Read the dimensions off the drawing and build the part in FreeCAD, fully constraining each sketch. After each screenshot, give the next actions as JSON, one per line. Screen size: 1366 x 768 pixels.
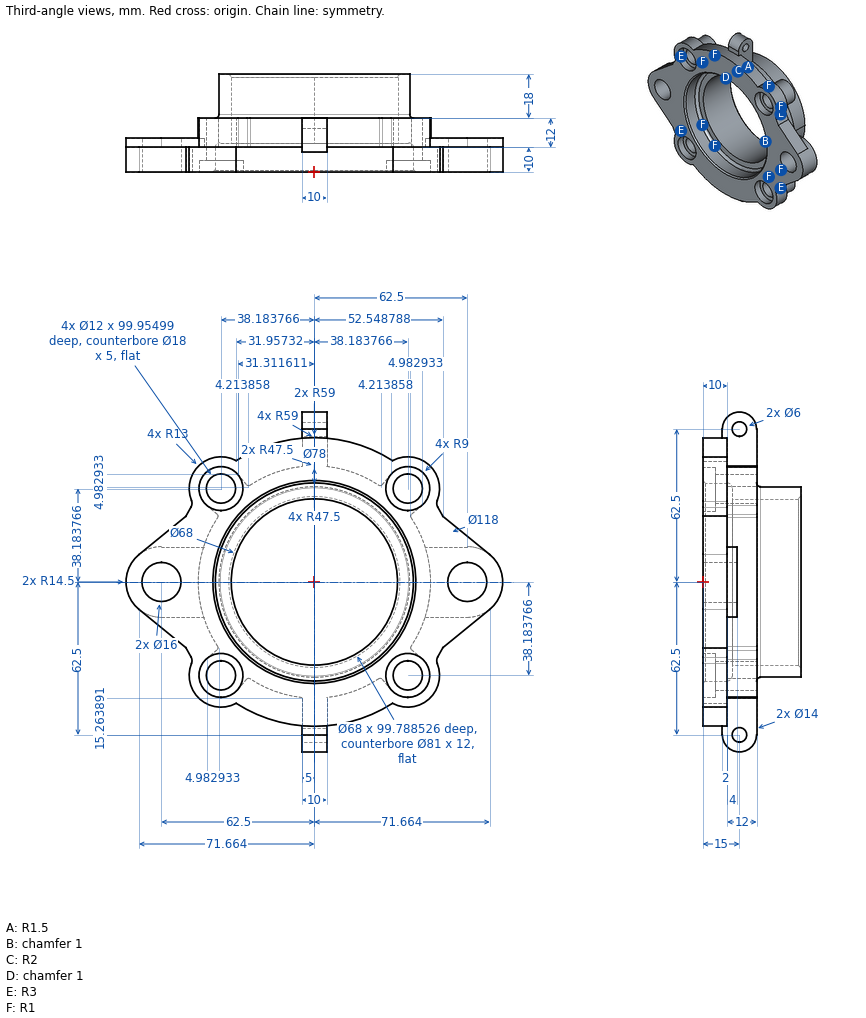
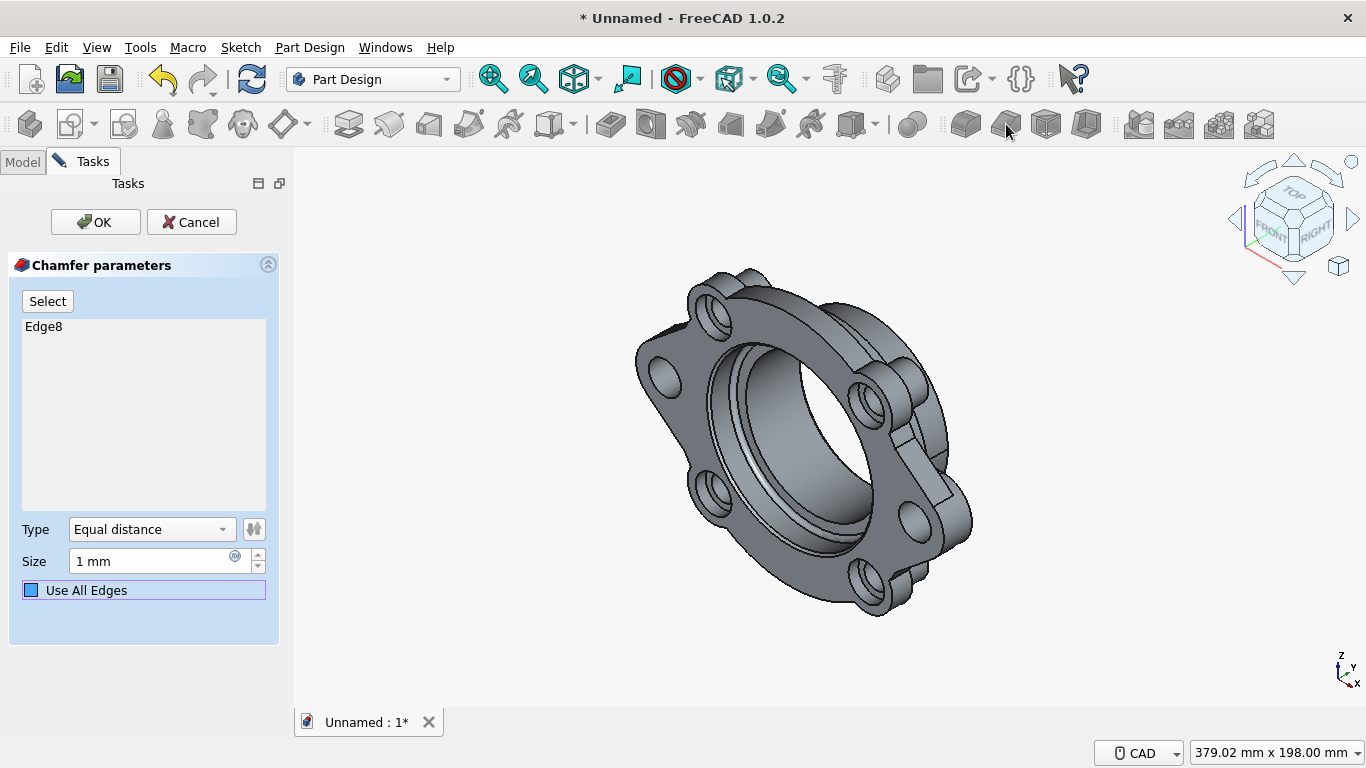
{"action": "left_click", "coordinate": [96, 222]}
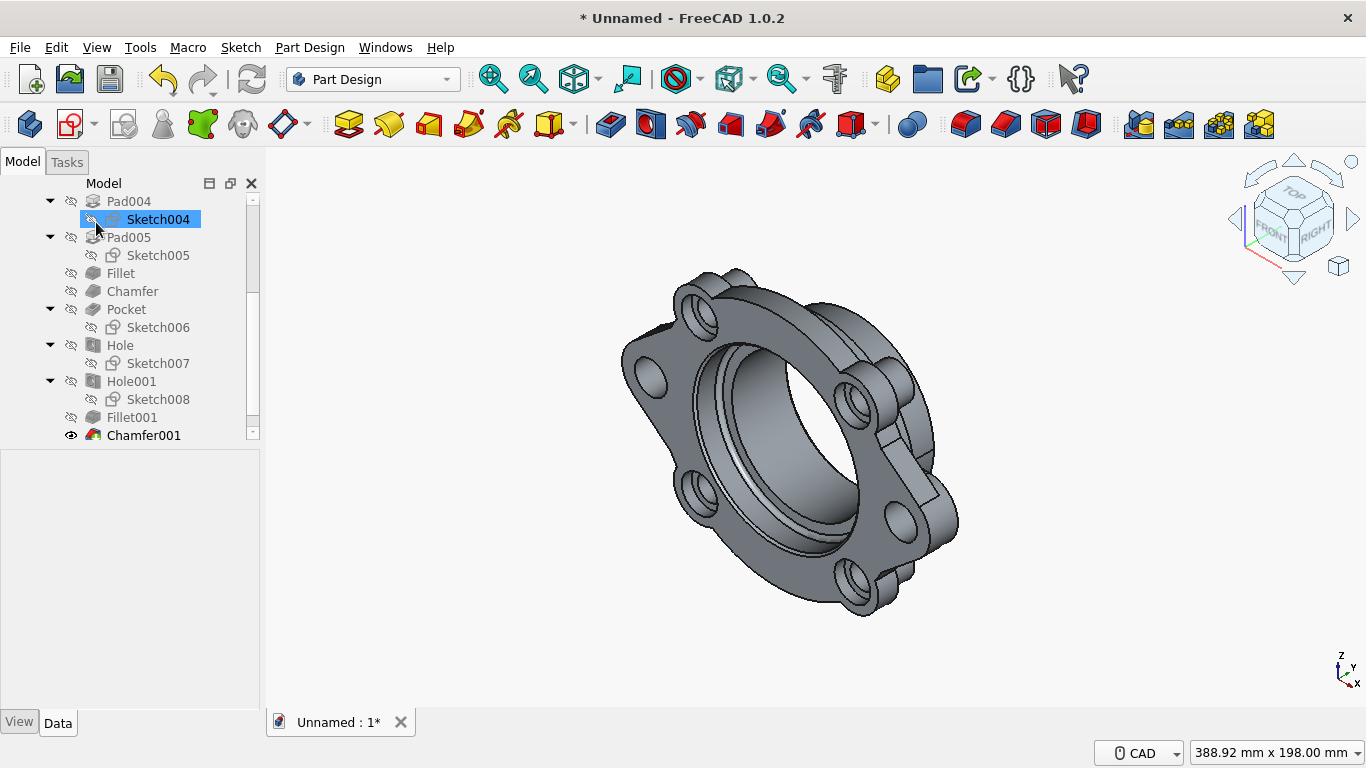
{"action": "key", "text": "4"}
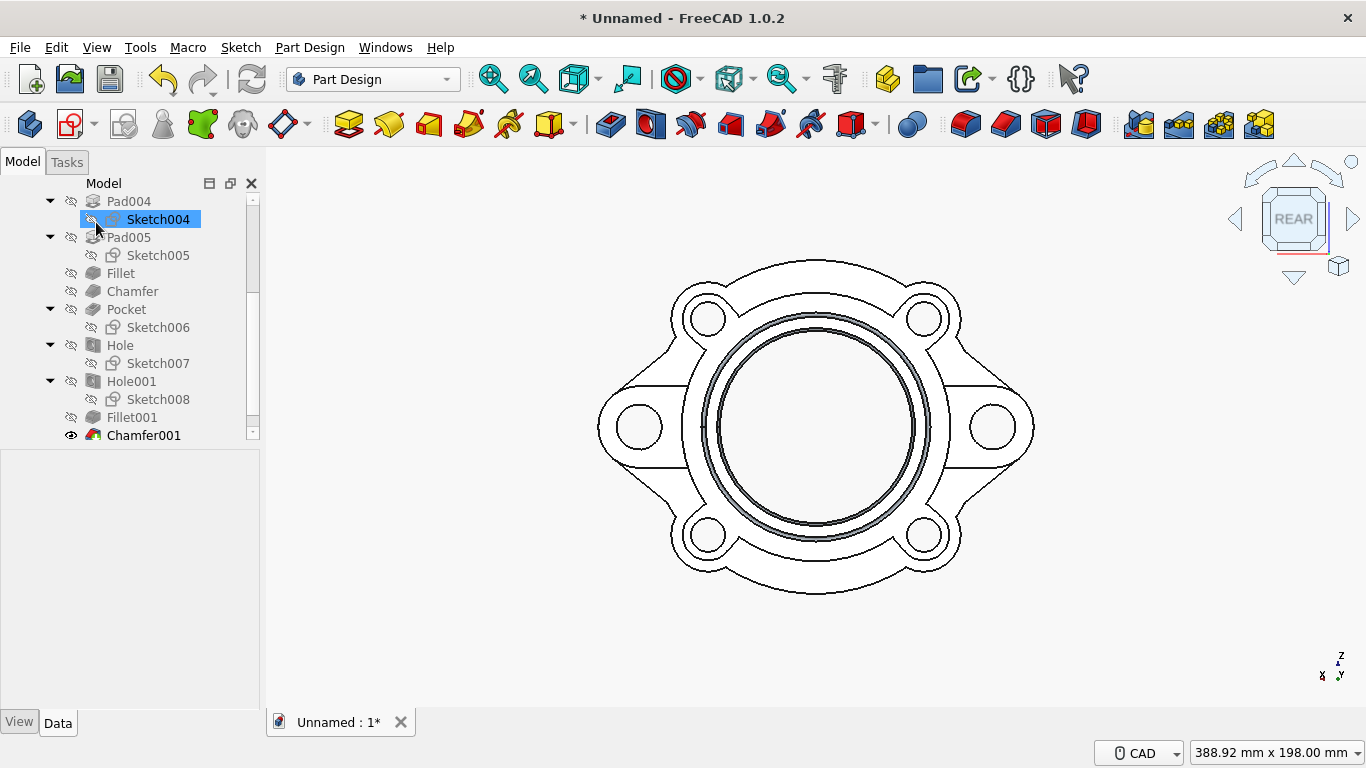
{"action": "left_click", "coordinate": [758, 288]}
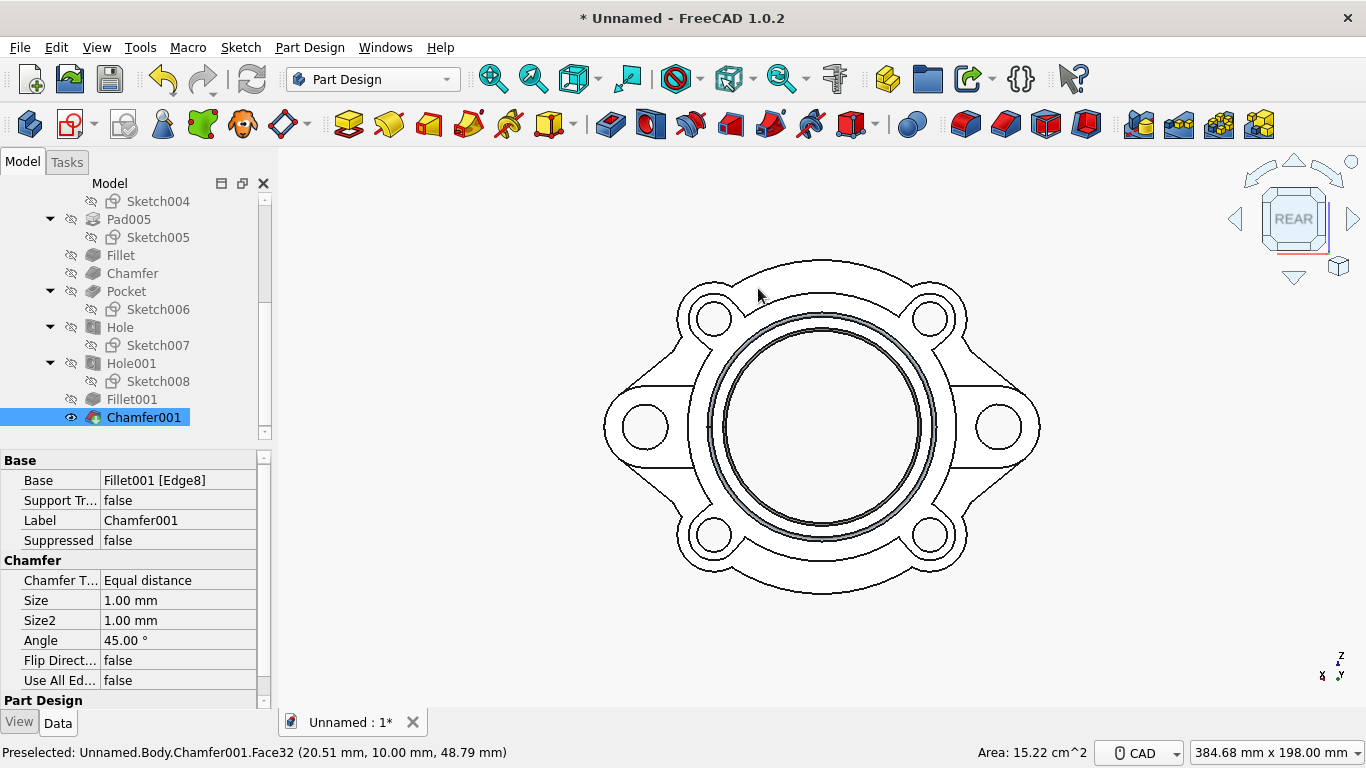
{"action": "left_click", "coordinate": [70, 124]}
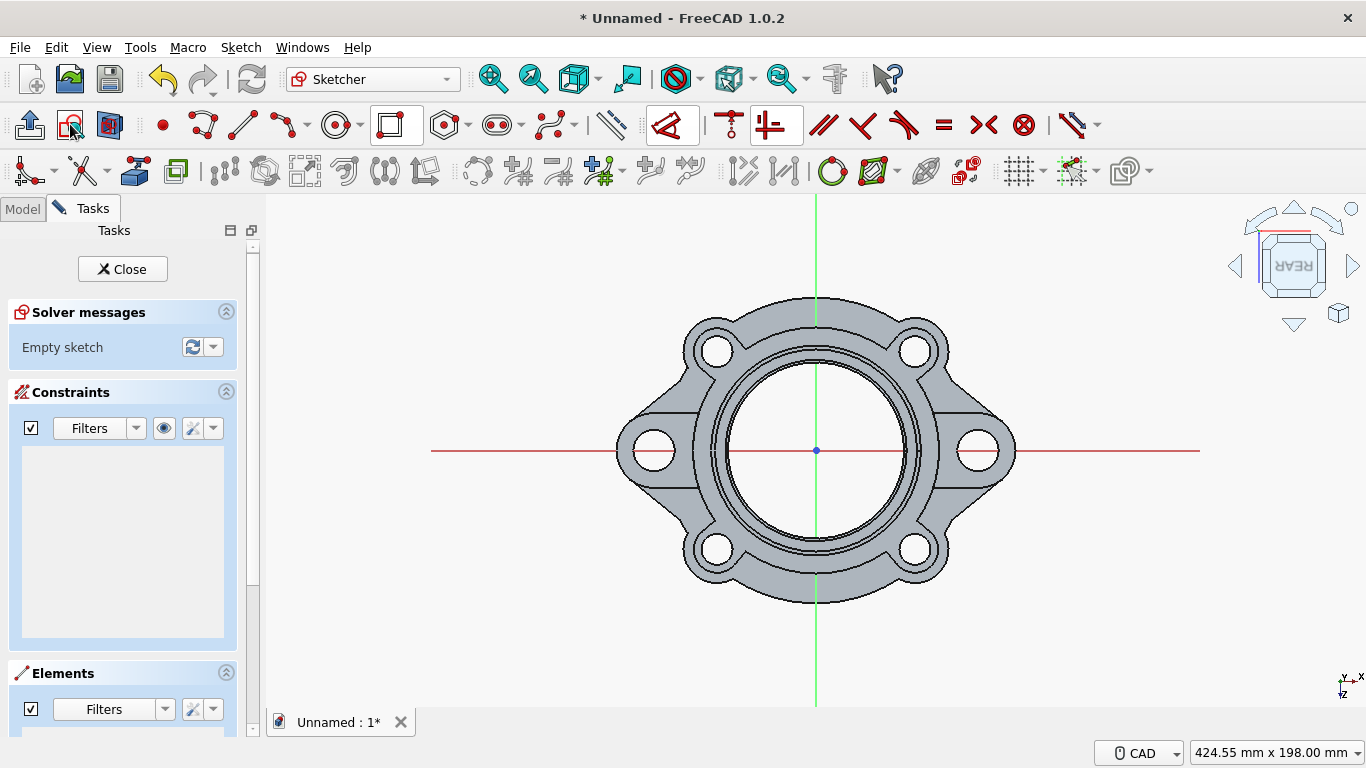
{"action": "left_click", "coordinate": [110, 126]}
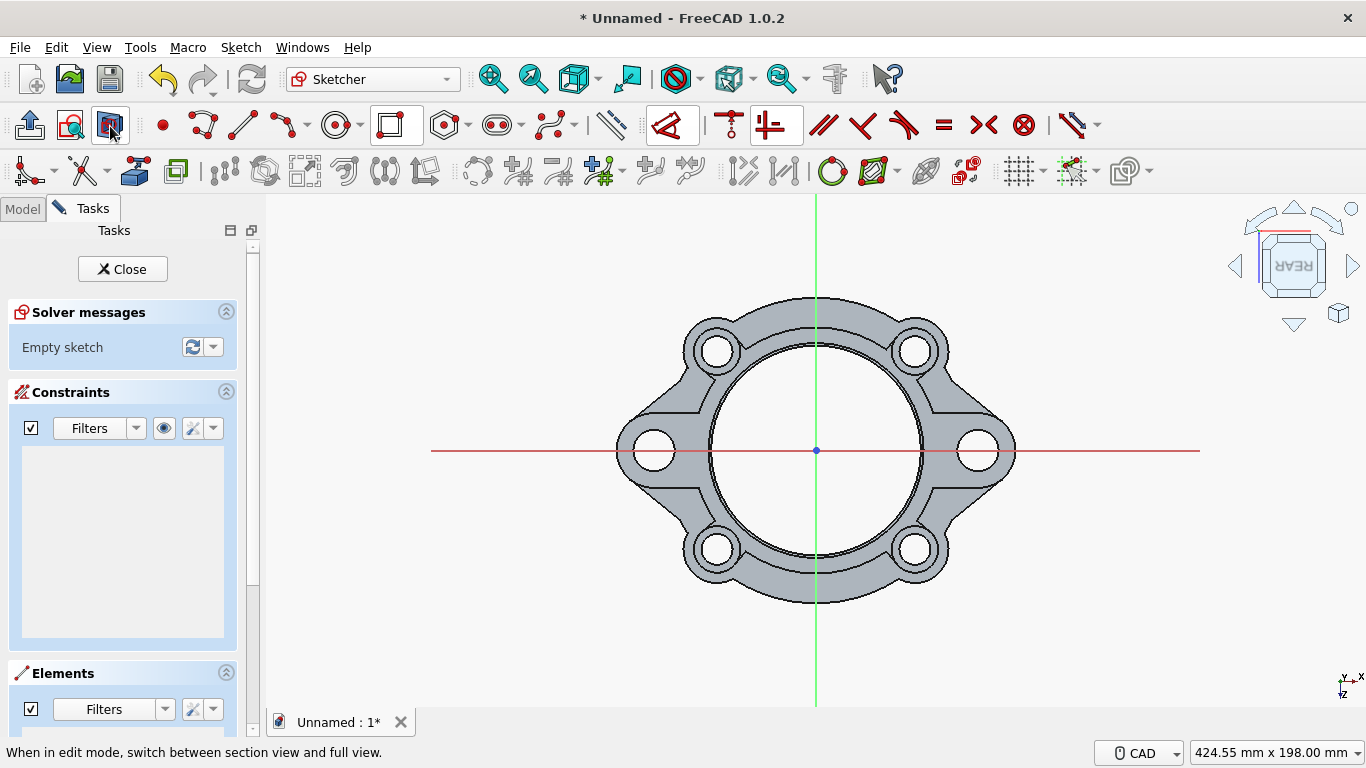
{"action": "left_click", "coordinate": [390, 126]}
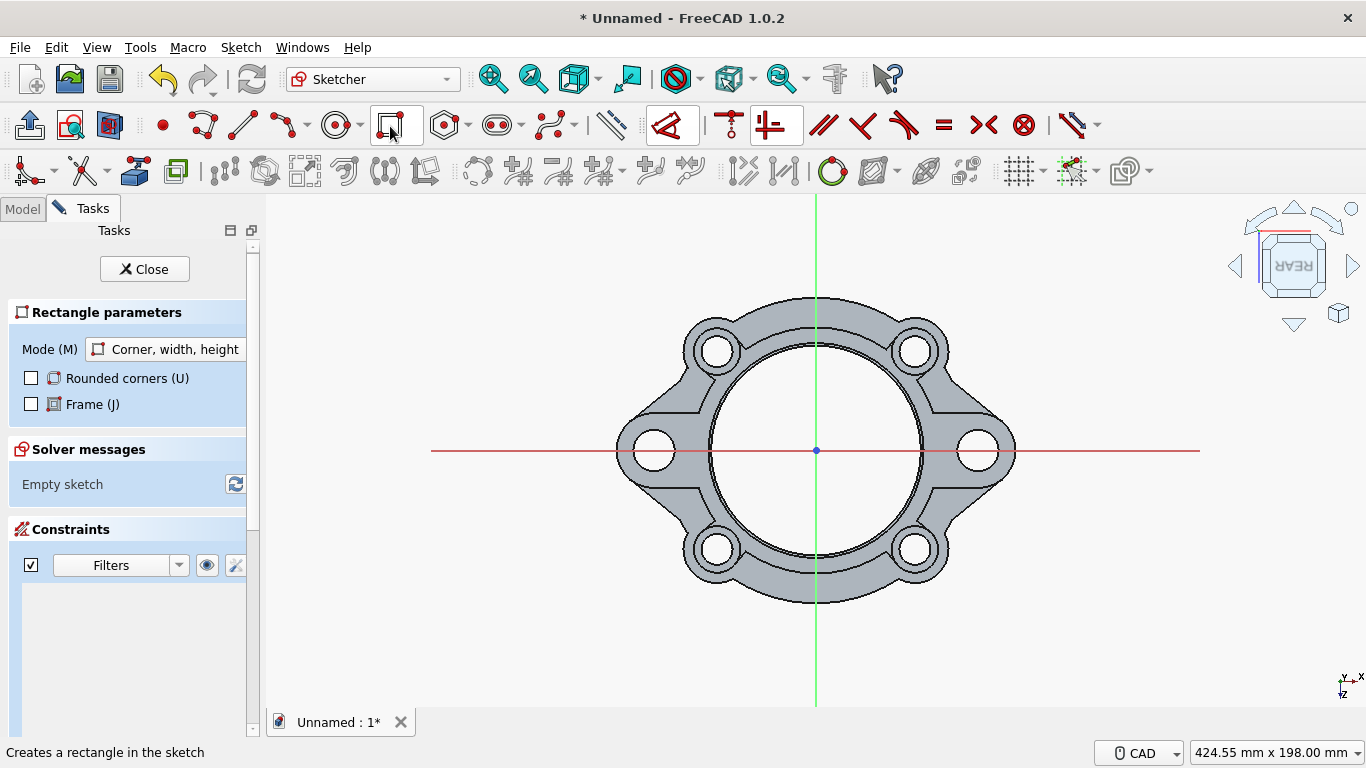
{"action": "scroll", "coordinate": [803, 289], "scroll_direction": "up", "scroll_amount": 2}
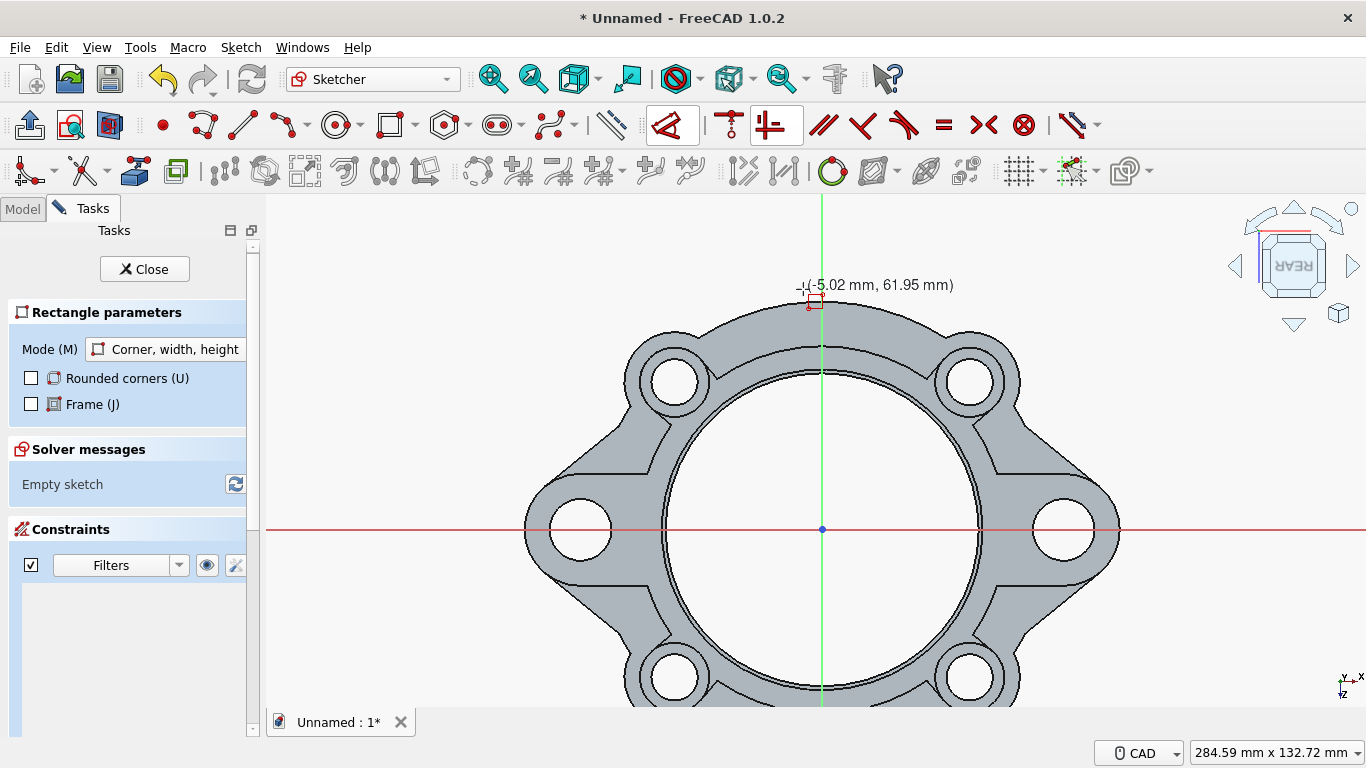
{"action": "left_click", "coordinate": [803, 288]}
{"action": "left_click", "coordinate": [841, 347]}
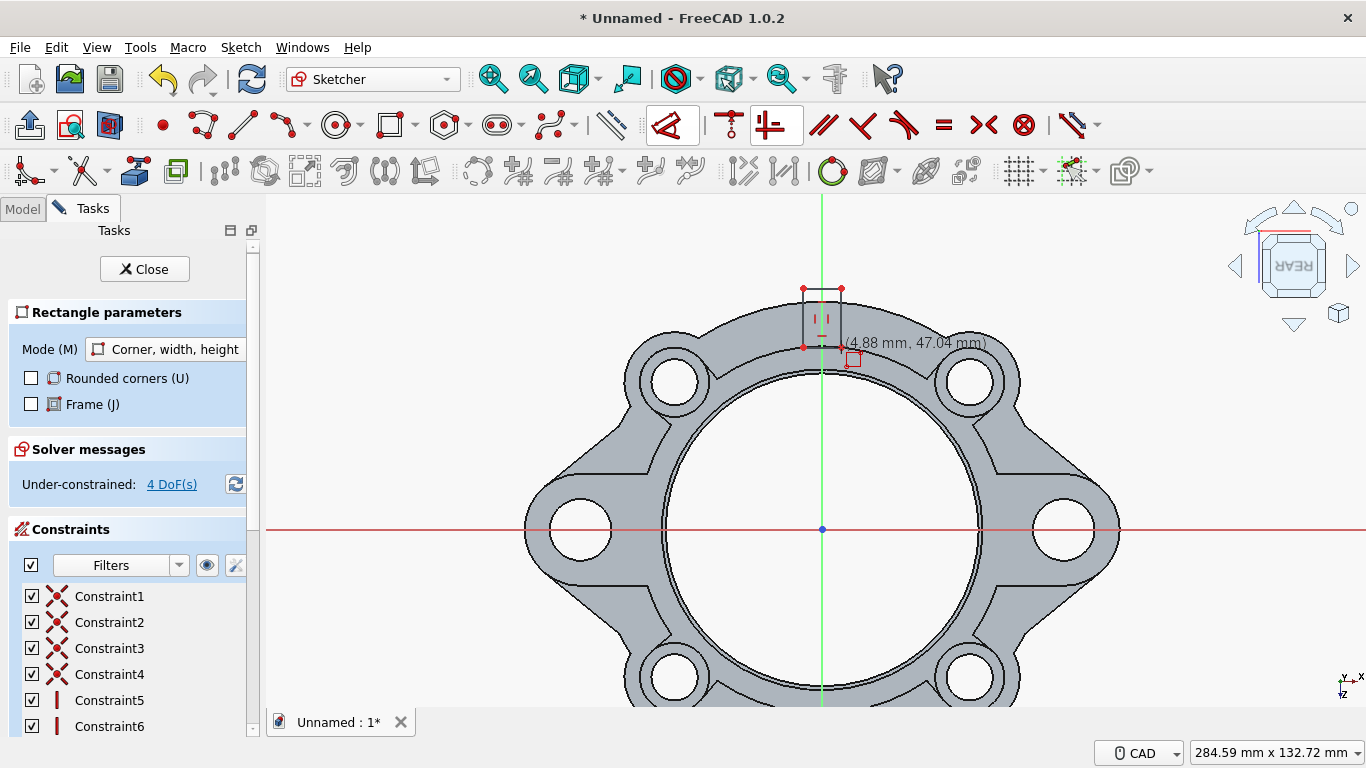
{"action": "scroll", "coordinate": [596, 289], "scroll_direction": "down", "scroll_amount": 2}